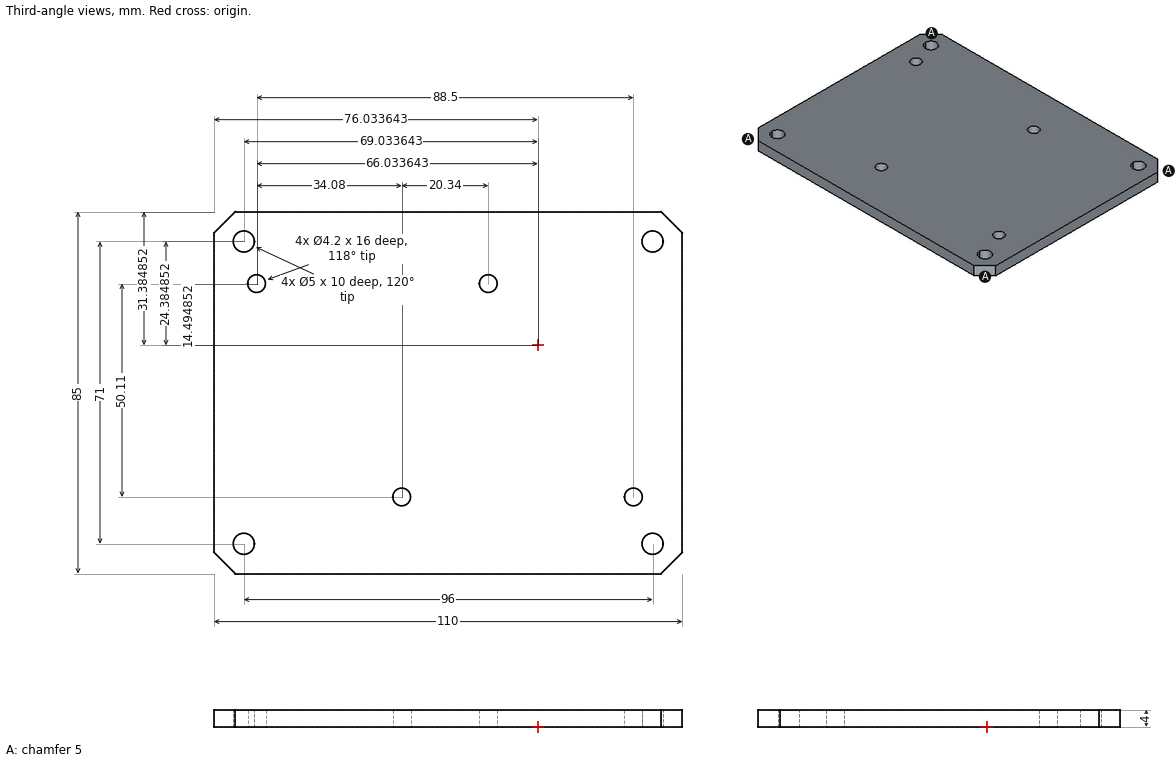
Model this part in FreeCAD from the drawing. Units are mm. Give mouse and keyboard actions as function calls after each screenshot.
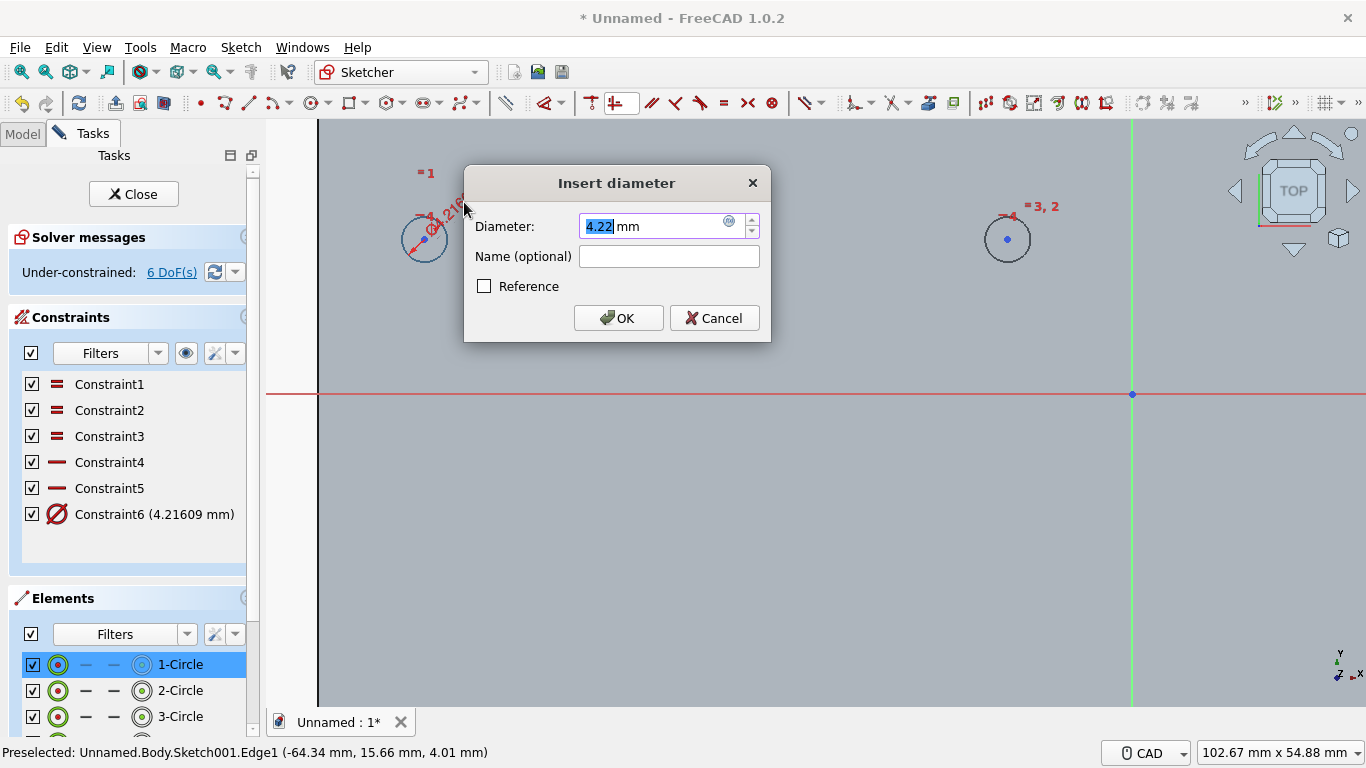
text(4.2)
key(Return)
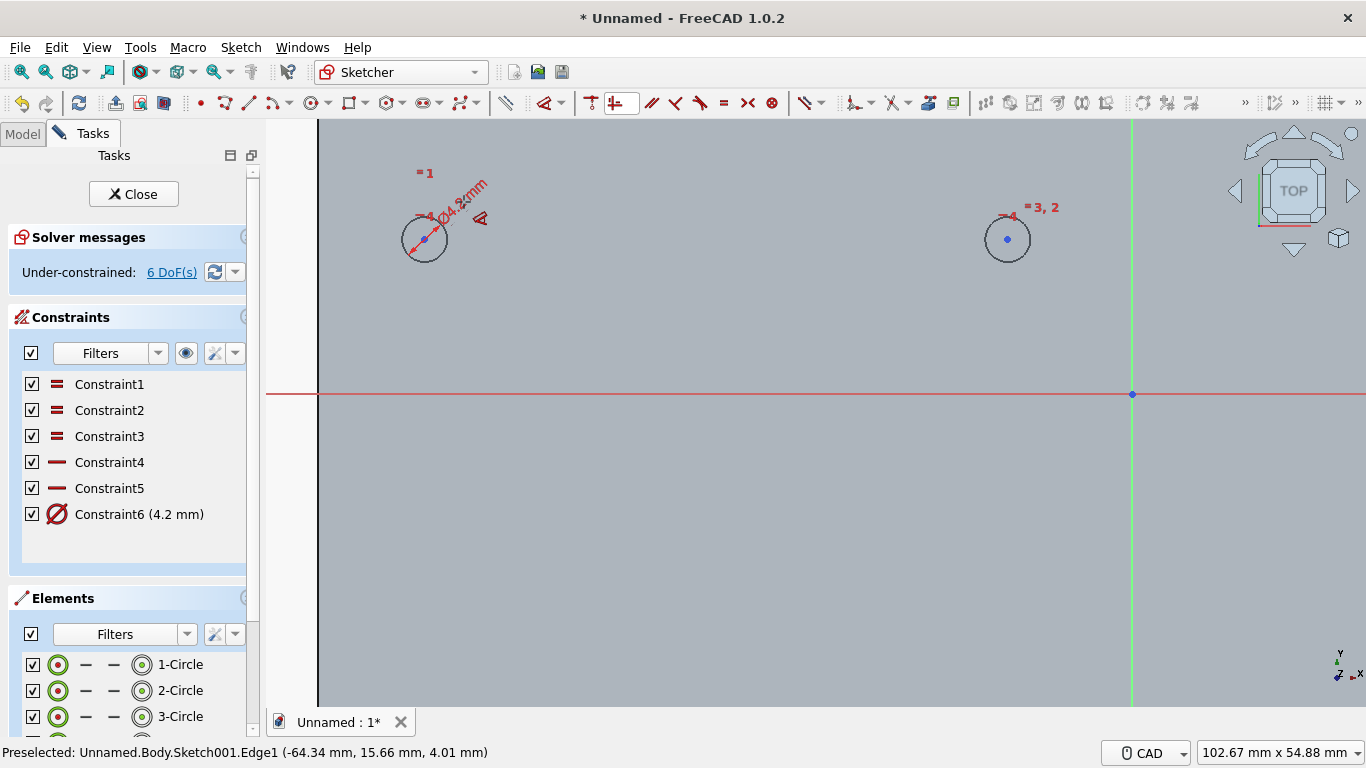
click(425, 240)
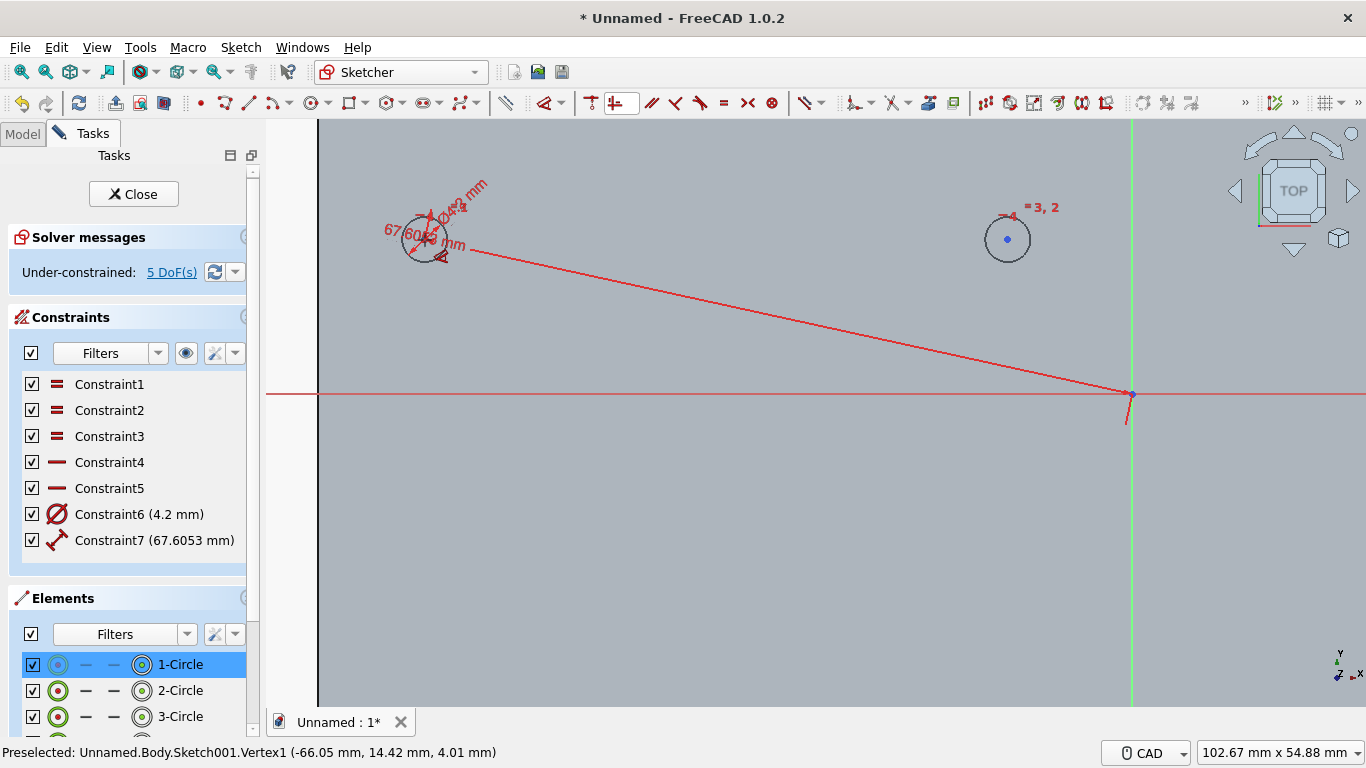
scroll(440, 221, down, 2)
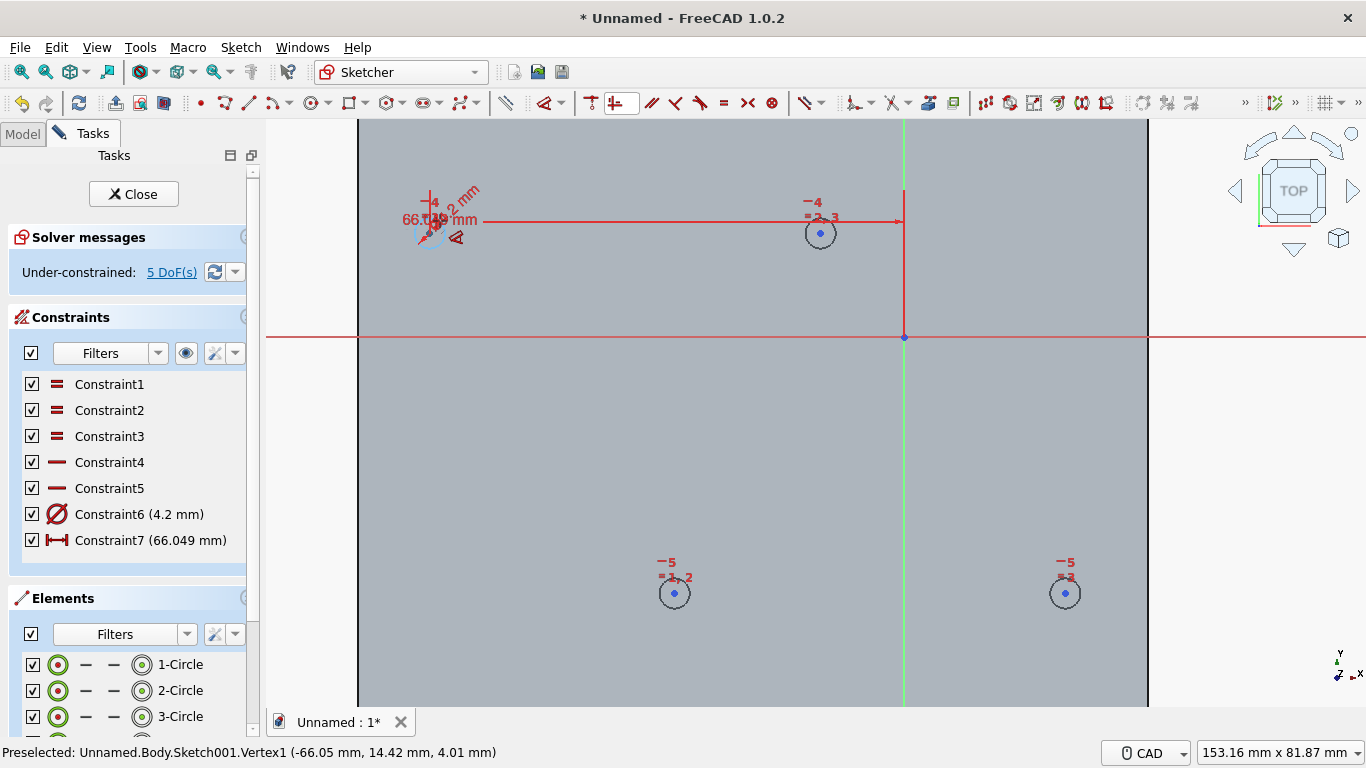
click(1065, 594)
click(748, 628)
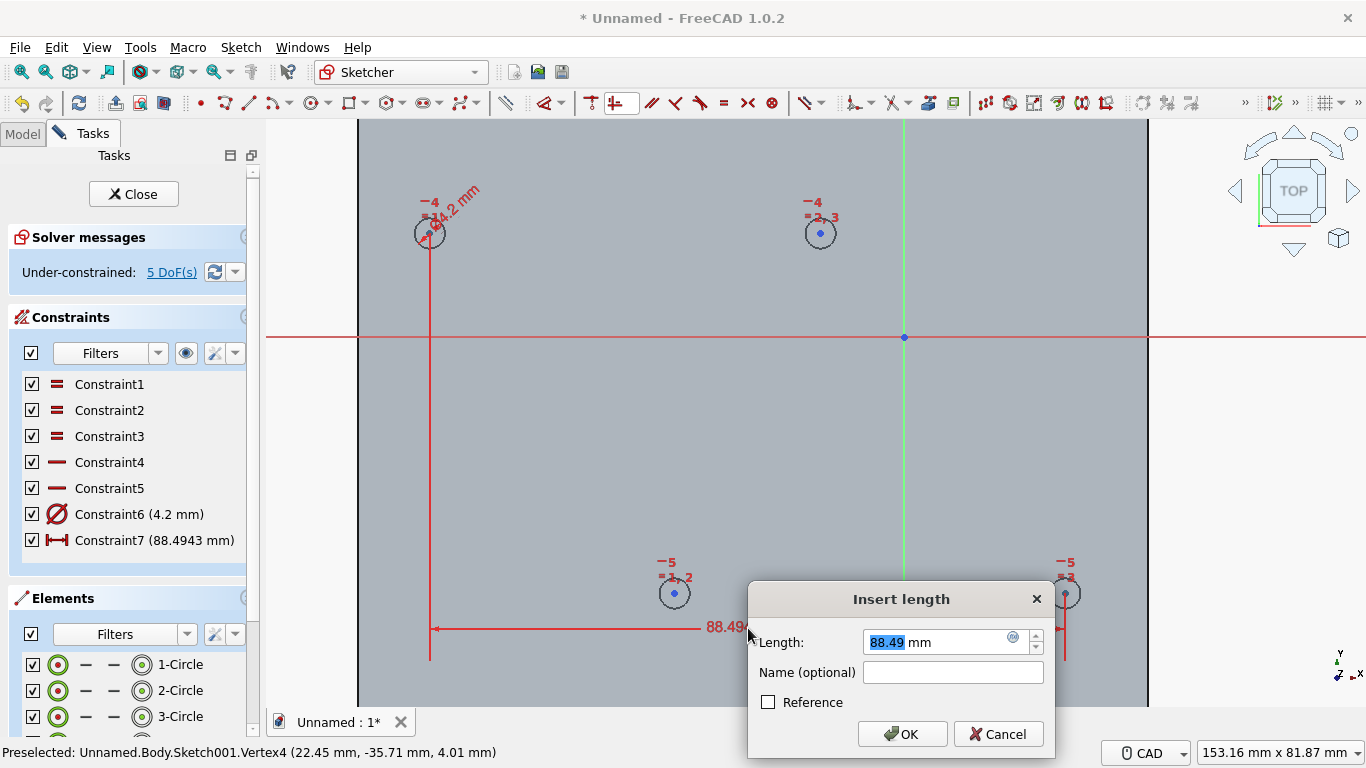
text(88.5)
key(Return)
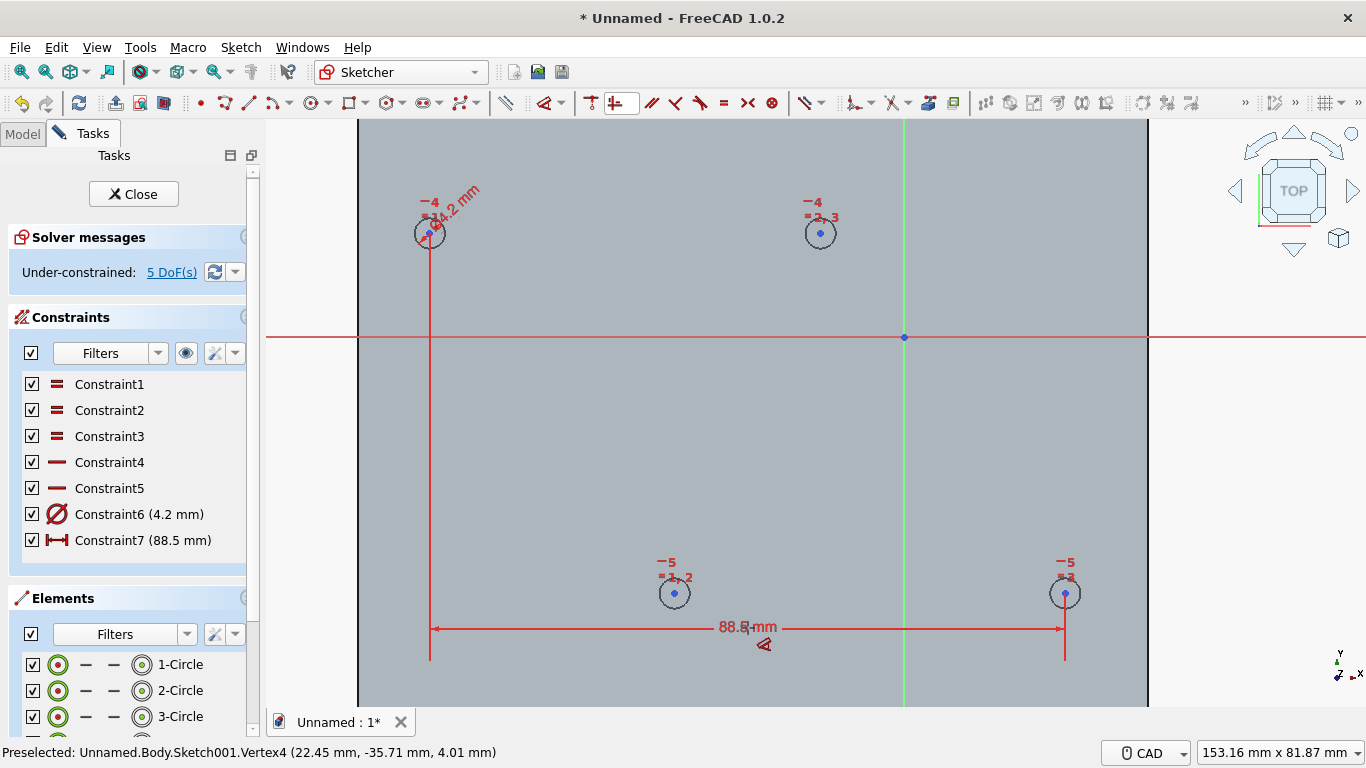
click(430, 233)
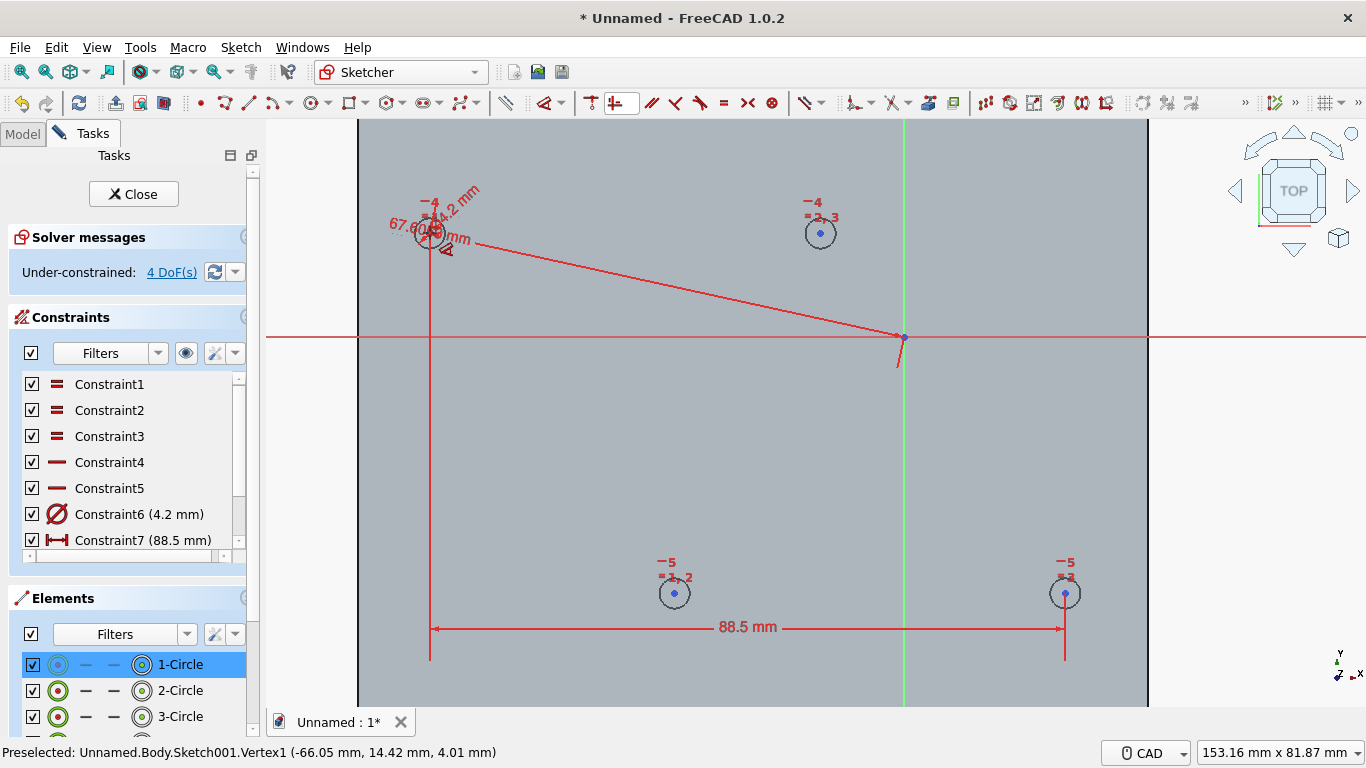
click(675, 594)
click(552, 628)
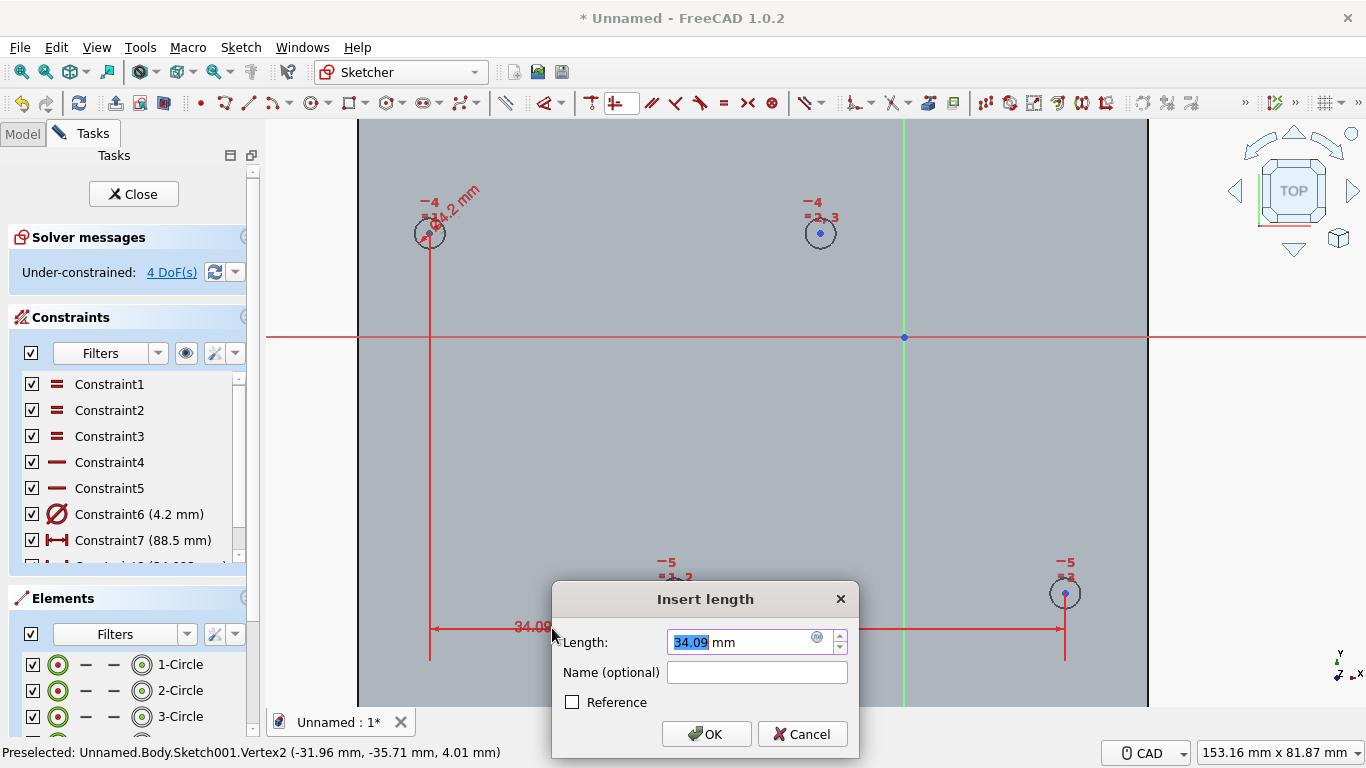
text(34.08)
key(Return)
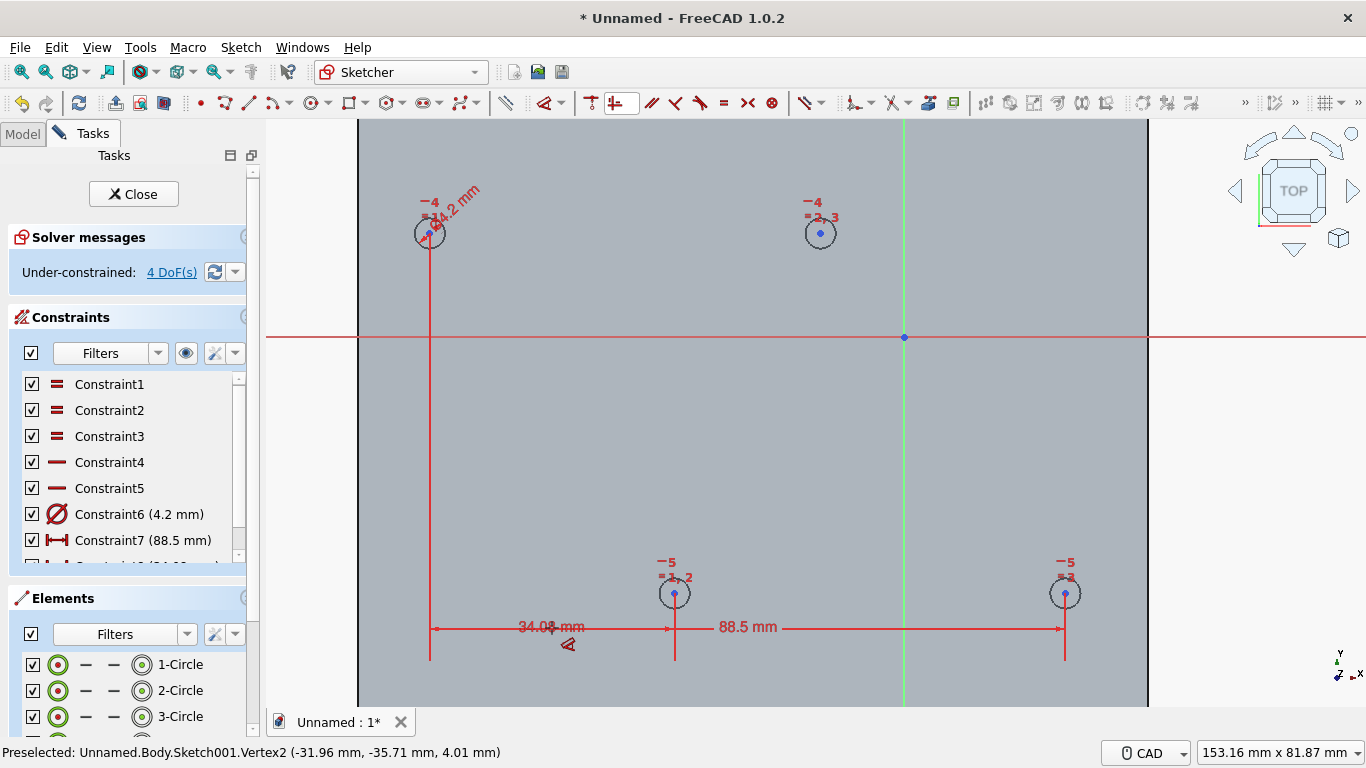
click(430, 233)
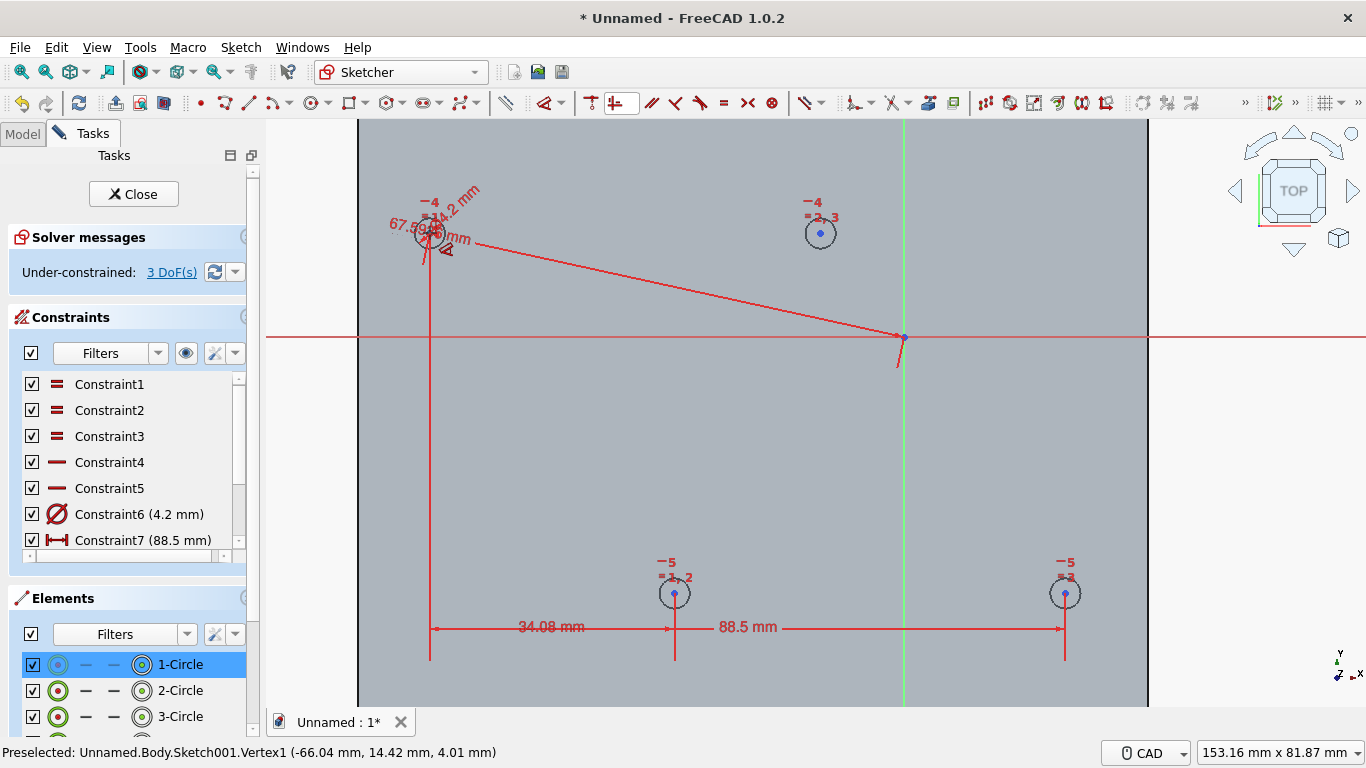
click(675, 594)
click(396, 414)